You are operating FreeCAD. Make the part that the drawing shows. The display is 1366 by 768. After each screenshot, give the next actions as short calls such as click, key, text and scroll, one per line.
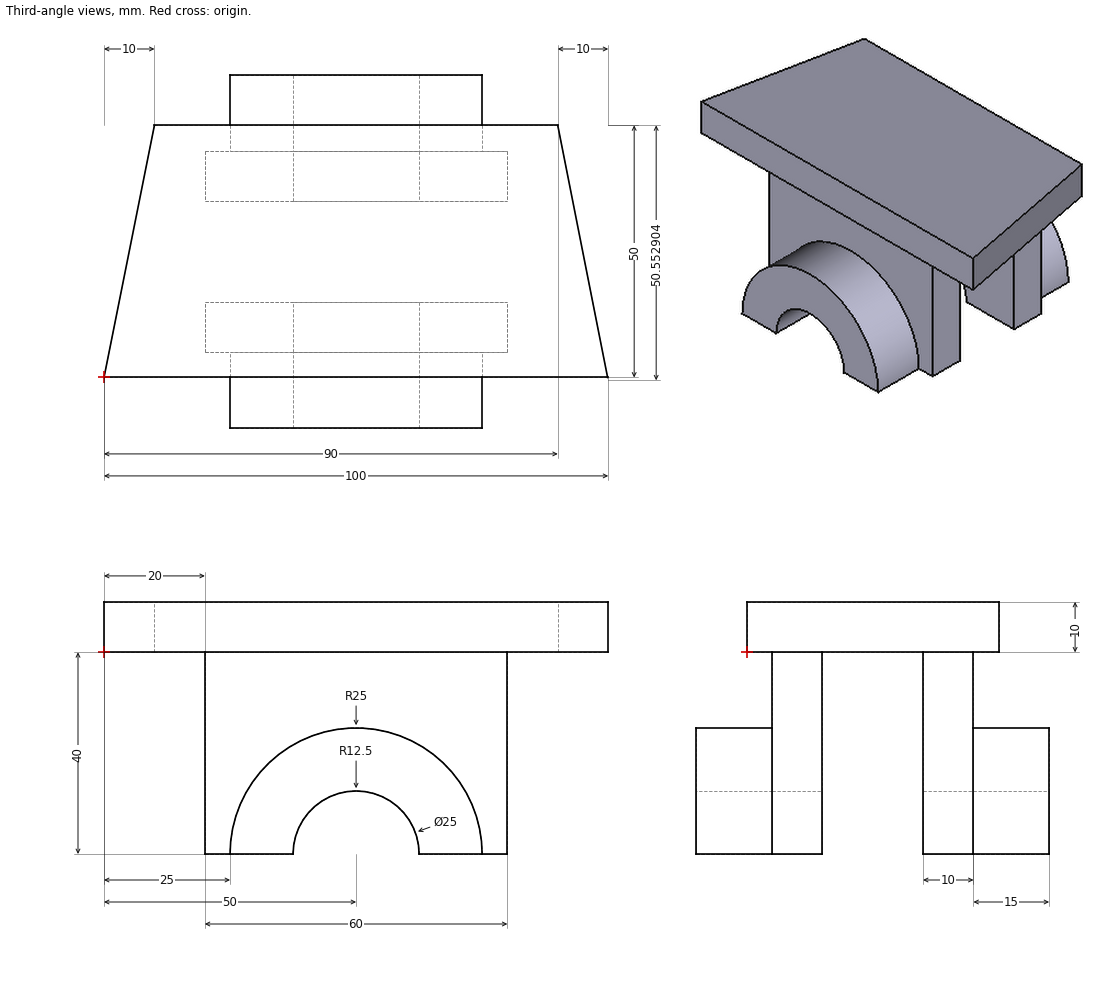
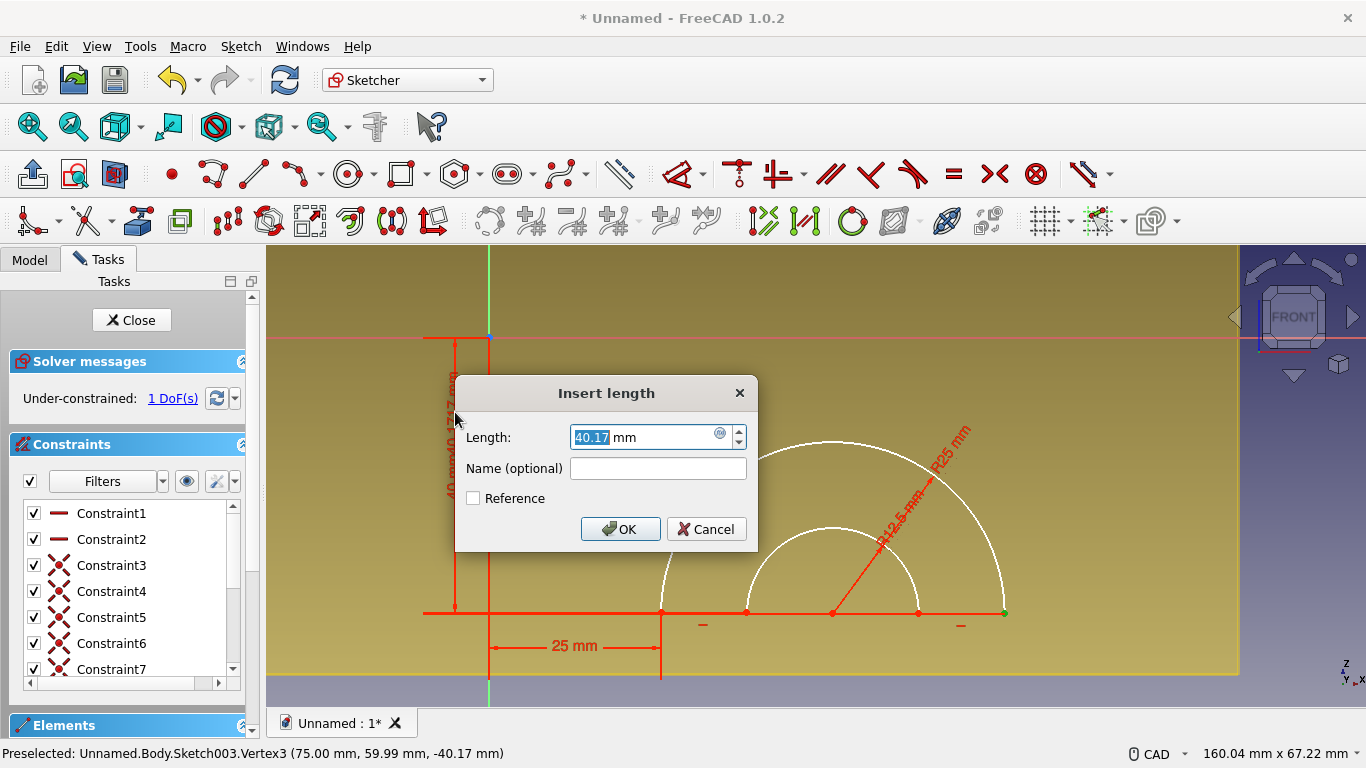
text(40)
key(Return)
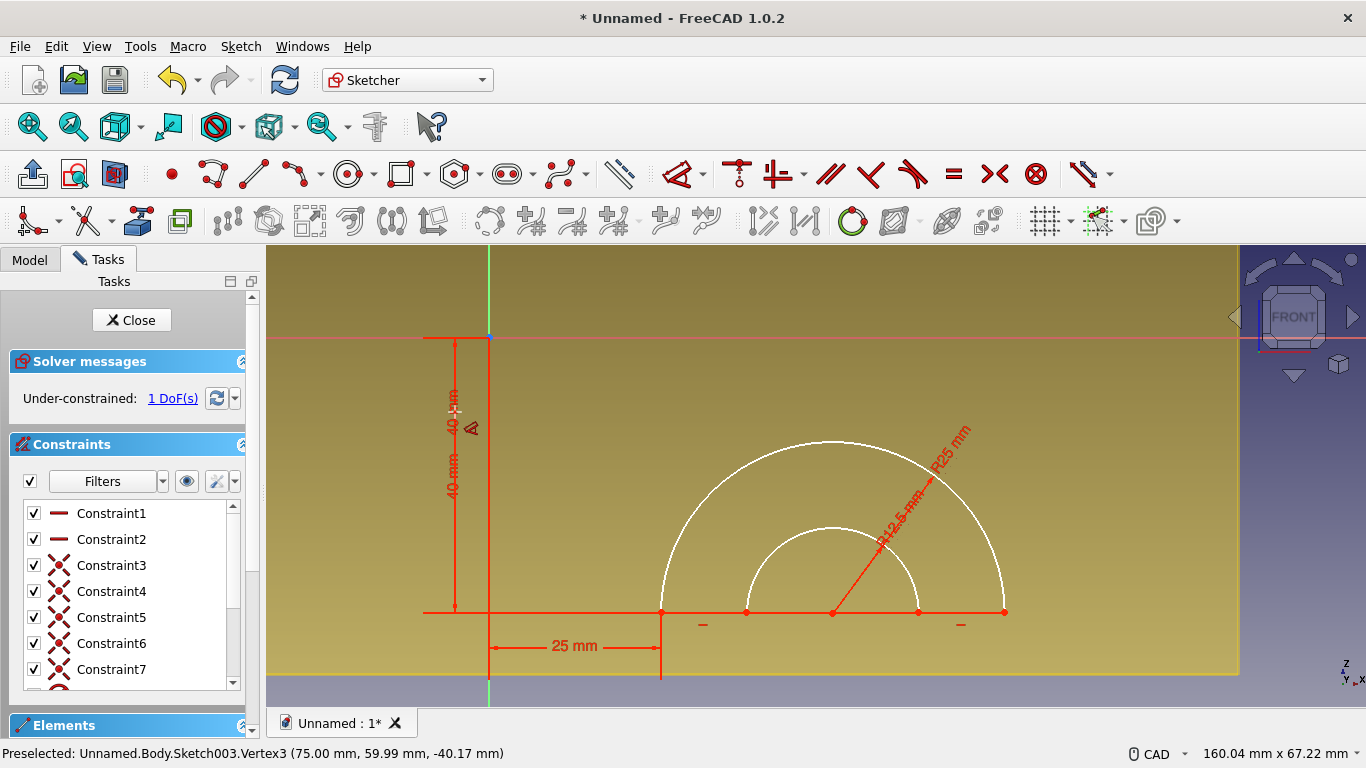
click(833, 614)
click(455, 539)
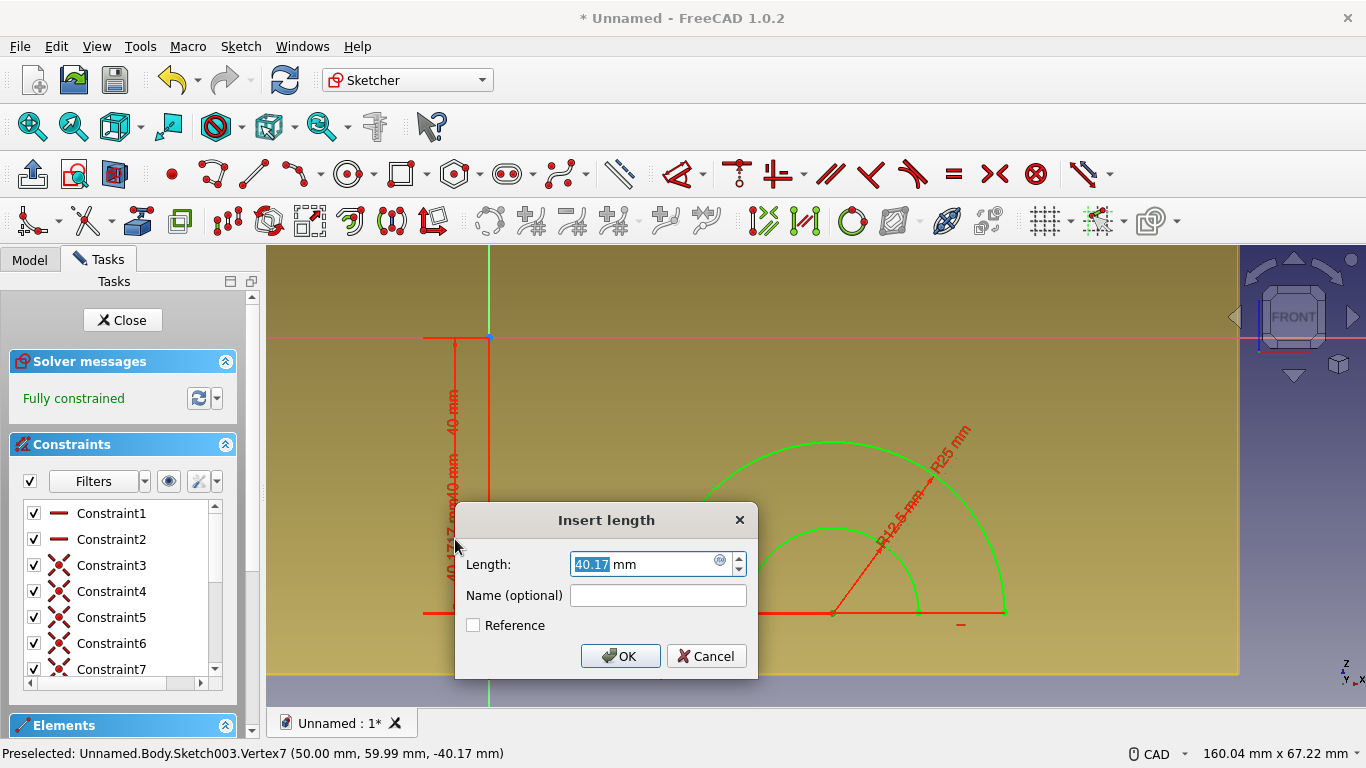
text(40)
key(Return)
key(Escape)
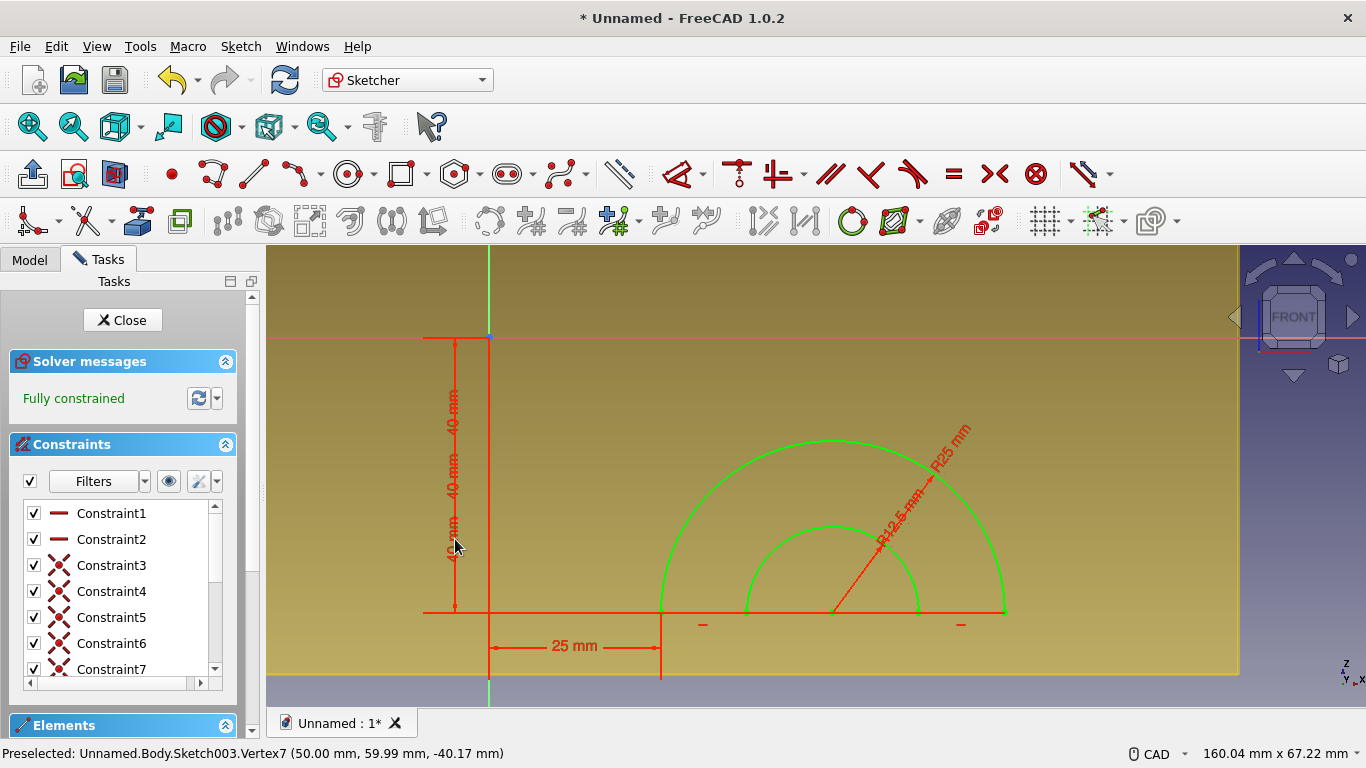
click(123, 320)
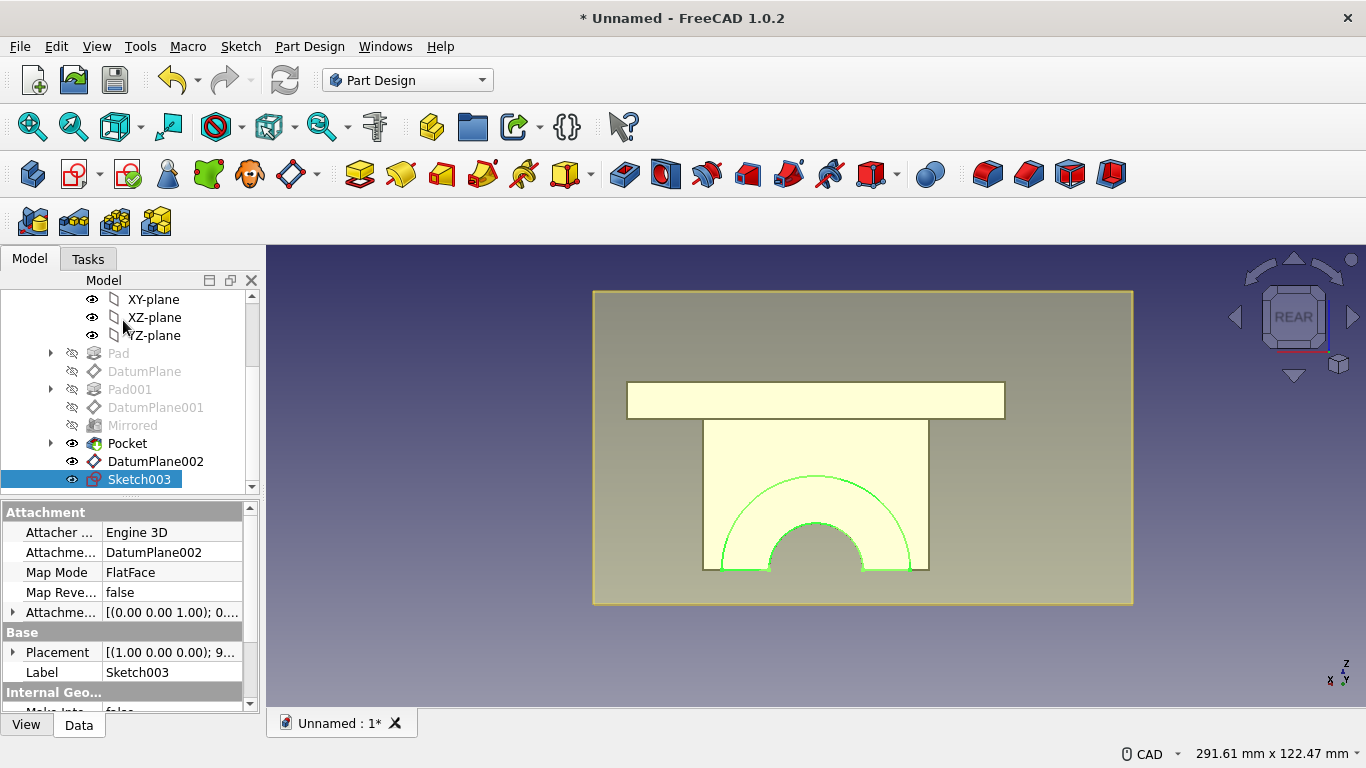
click(360, 174)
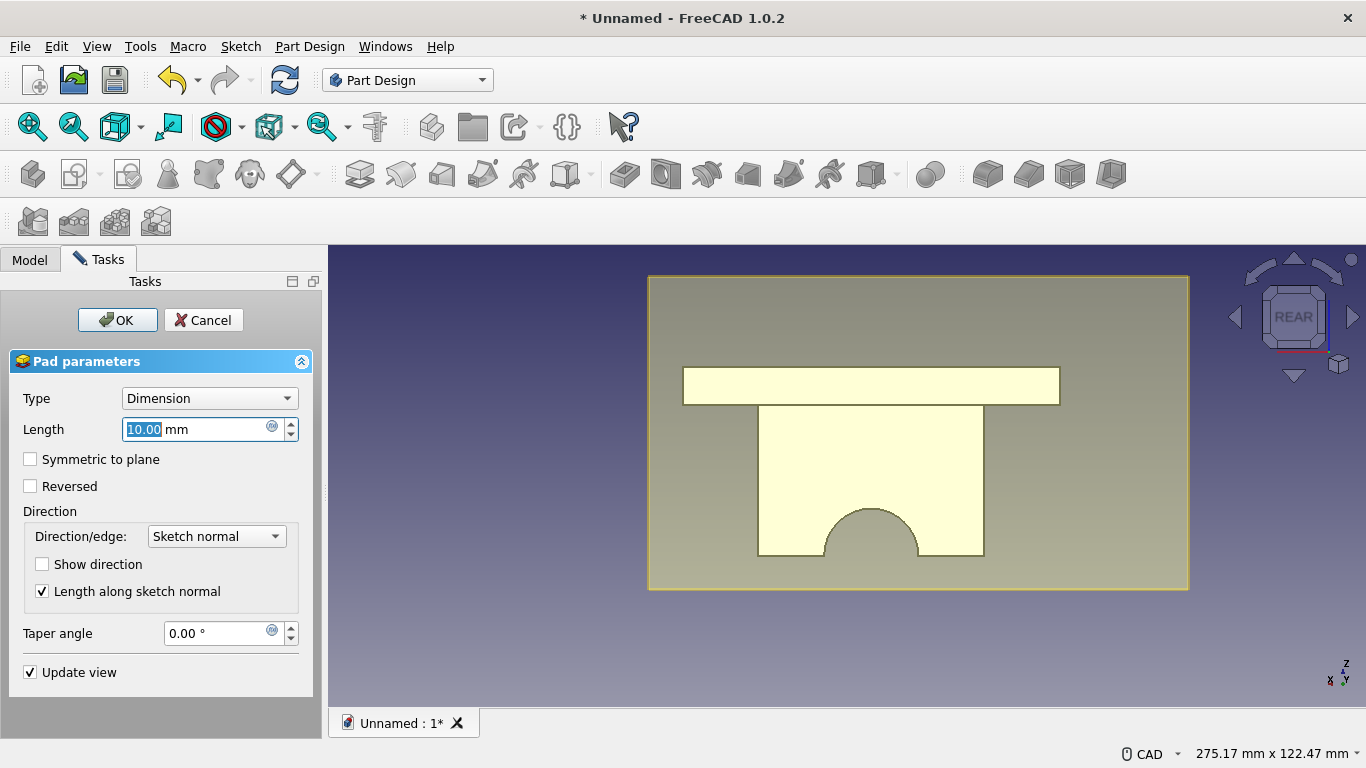
text(15)
key(Tab)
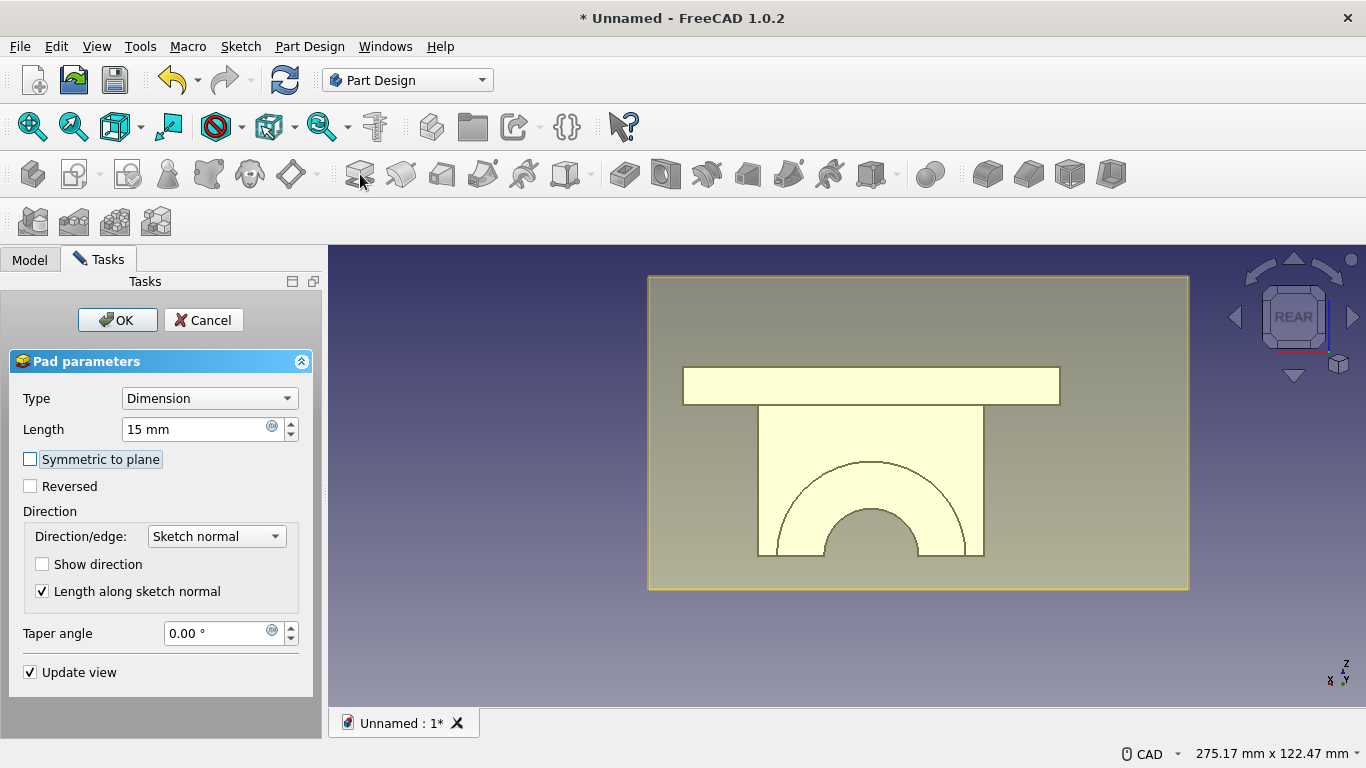
click(118, 320)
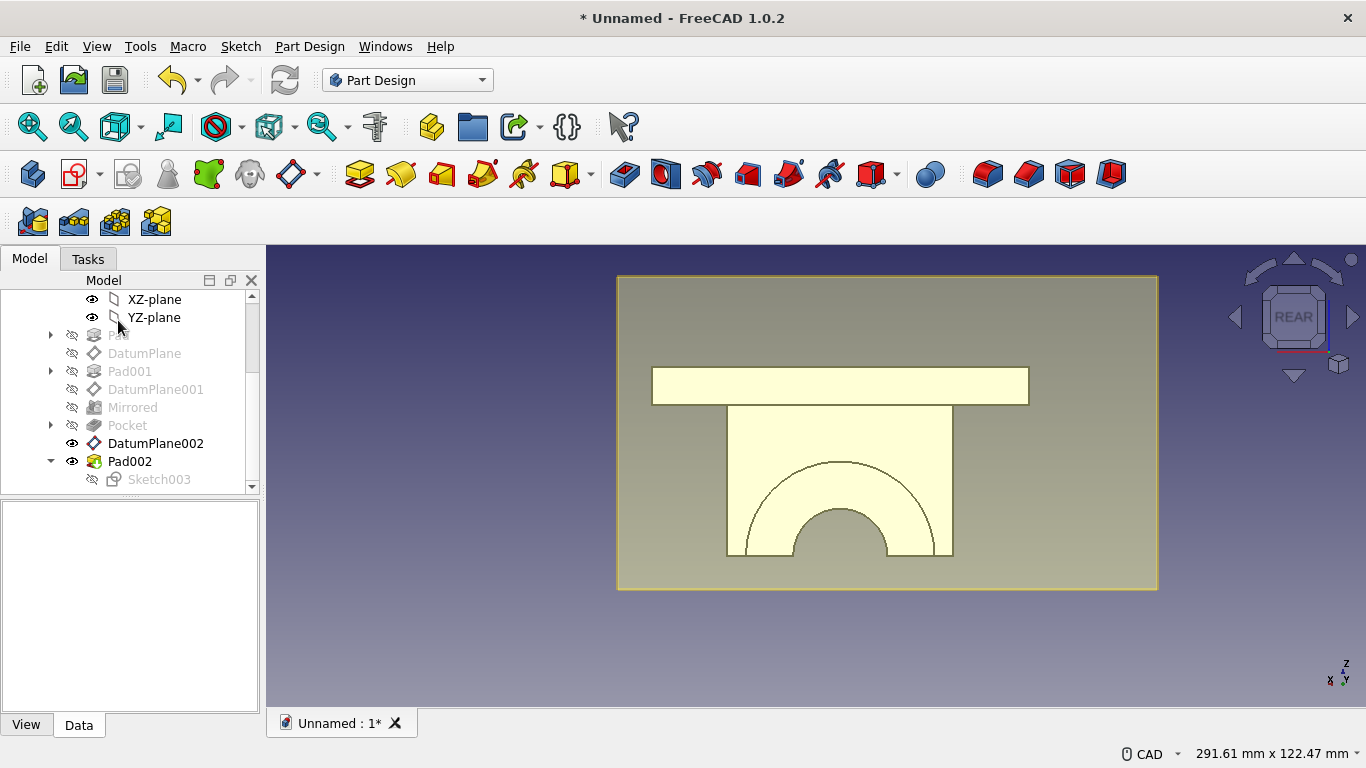
click(117, 443)
key(space)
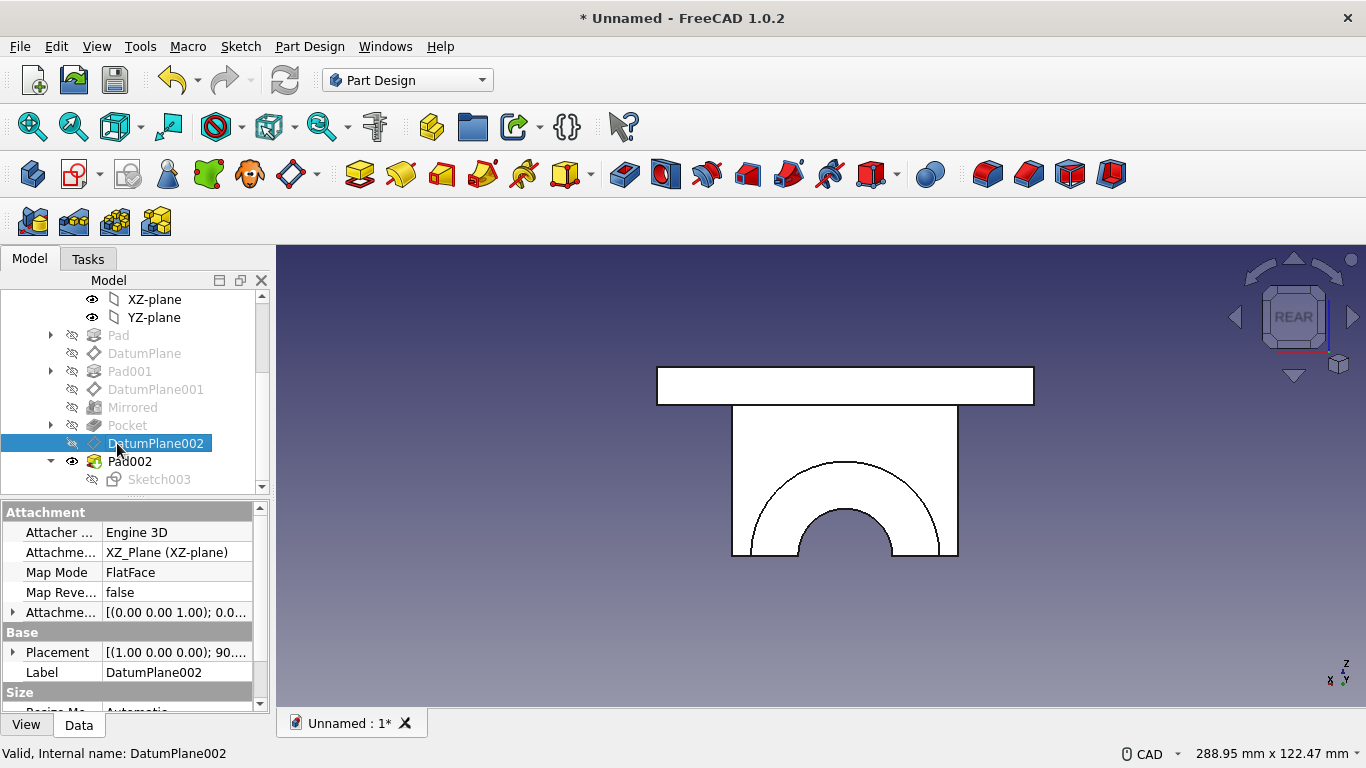
click(33, 128)